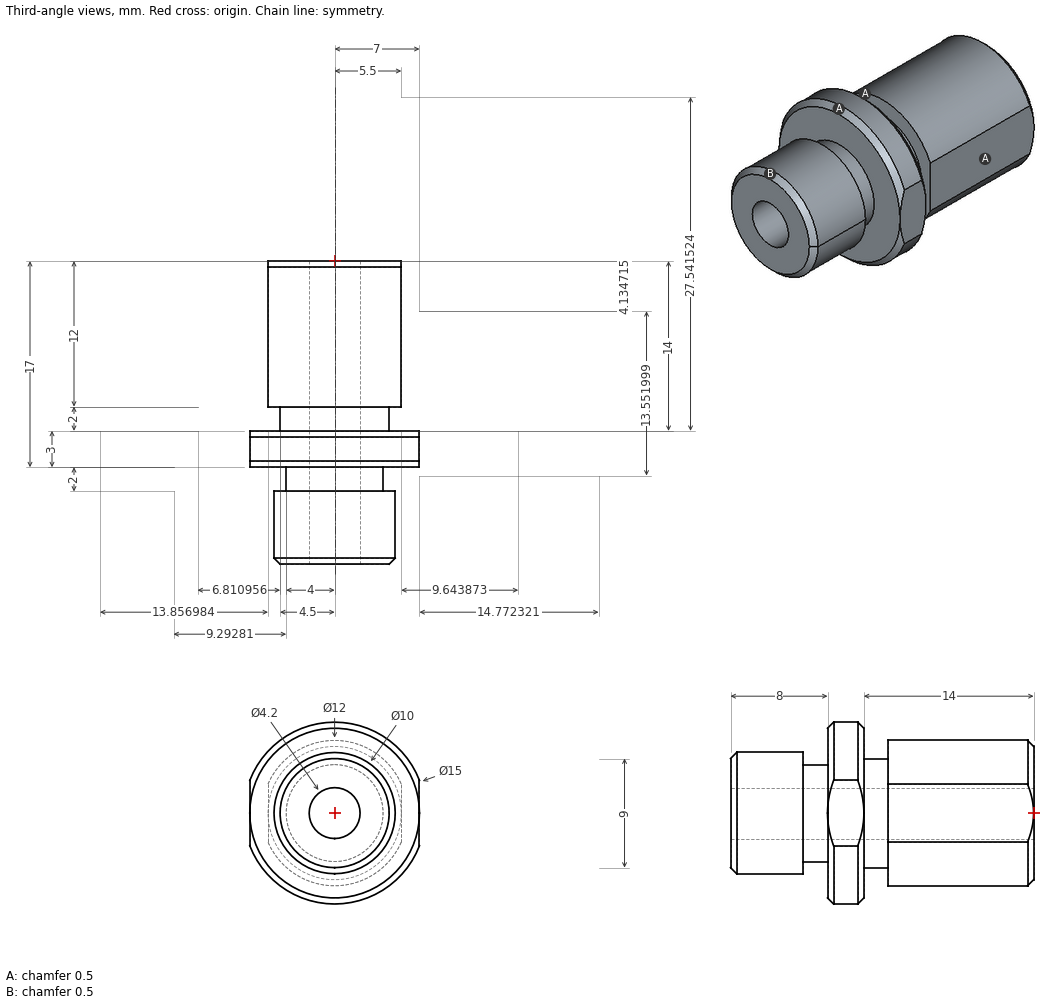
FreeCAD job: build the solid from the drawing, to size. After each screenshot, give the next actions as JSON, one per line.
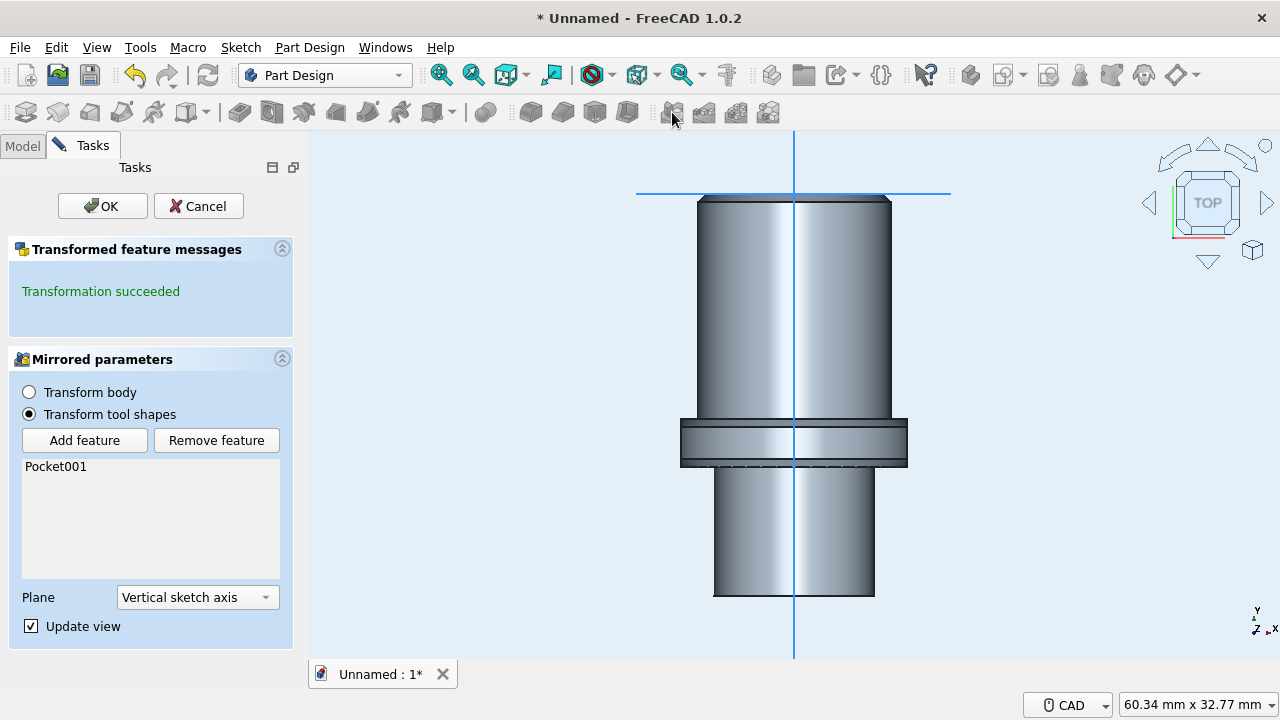
{"action": "left_click", "coordinate": [198, 598]}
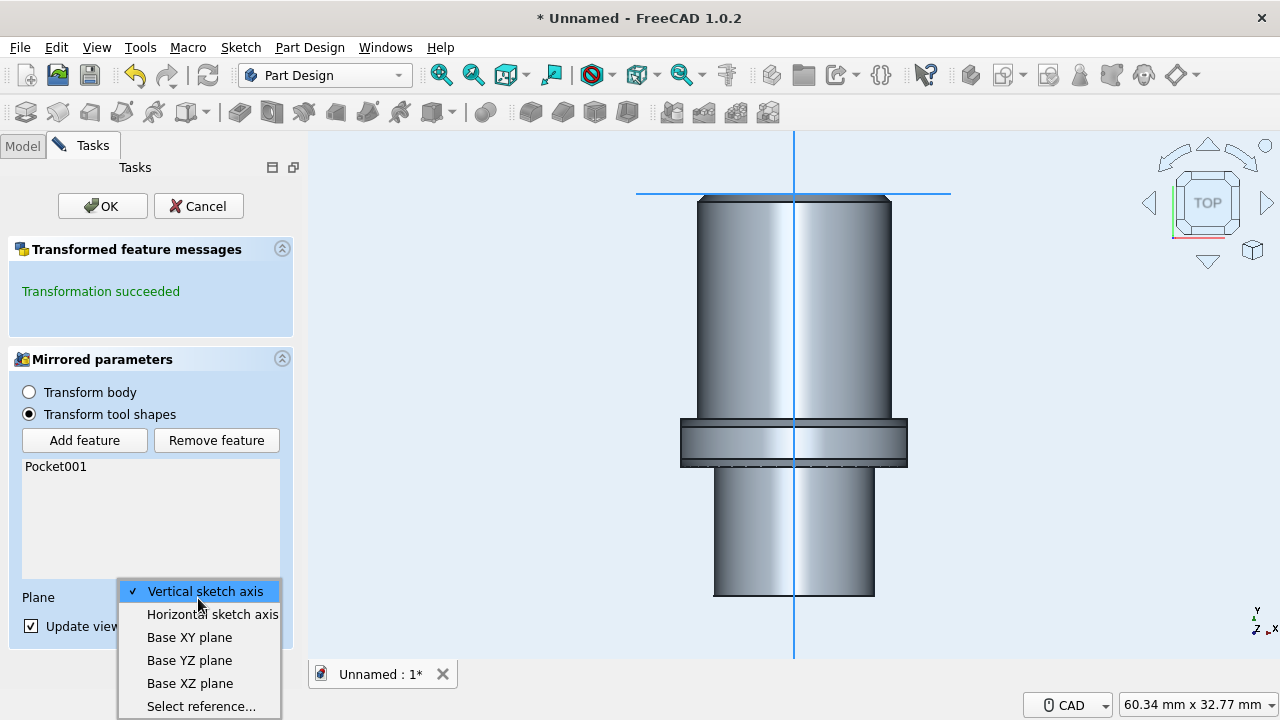
{"action": "left_click", "coordinate": [198, 660]}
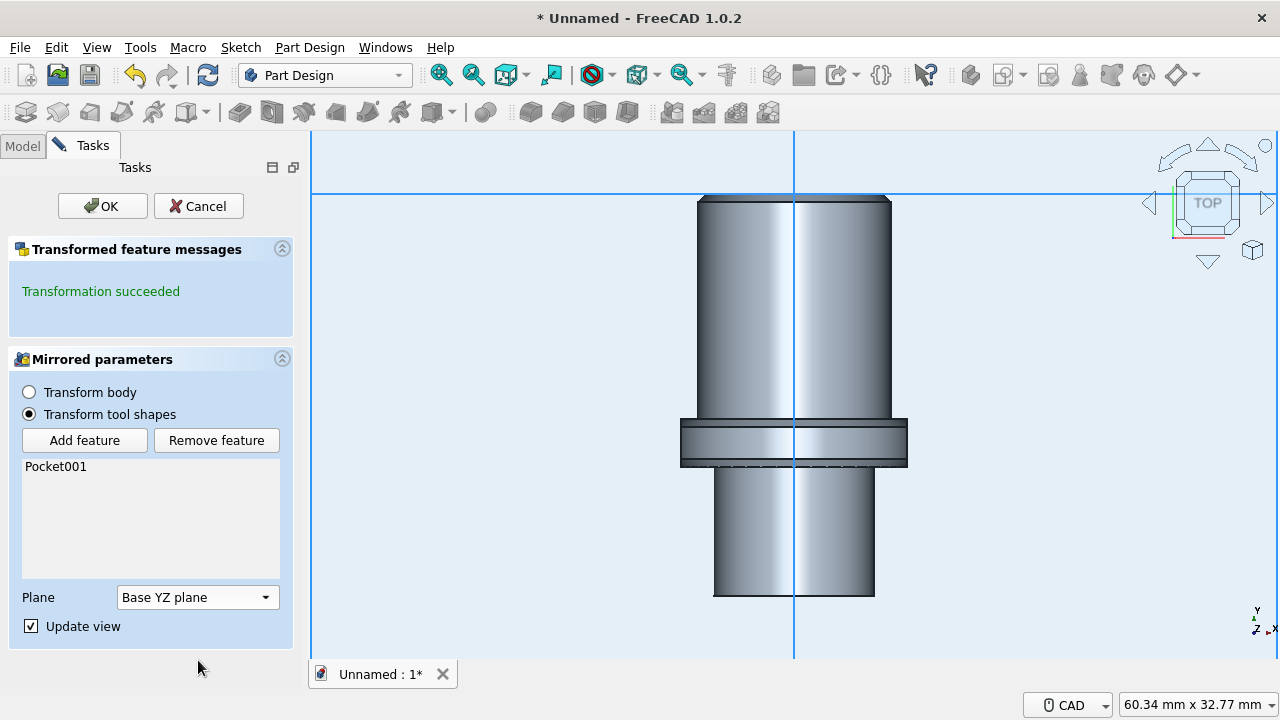
{"action": "left_click", "coordinate": [103, 206]}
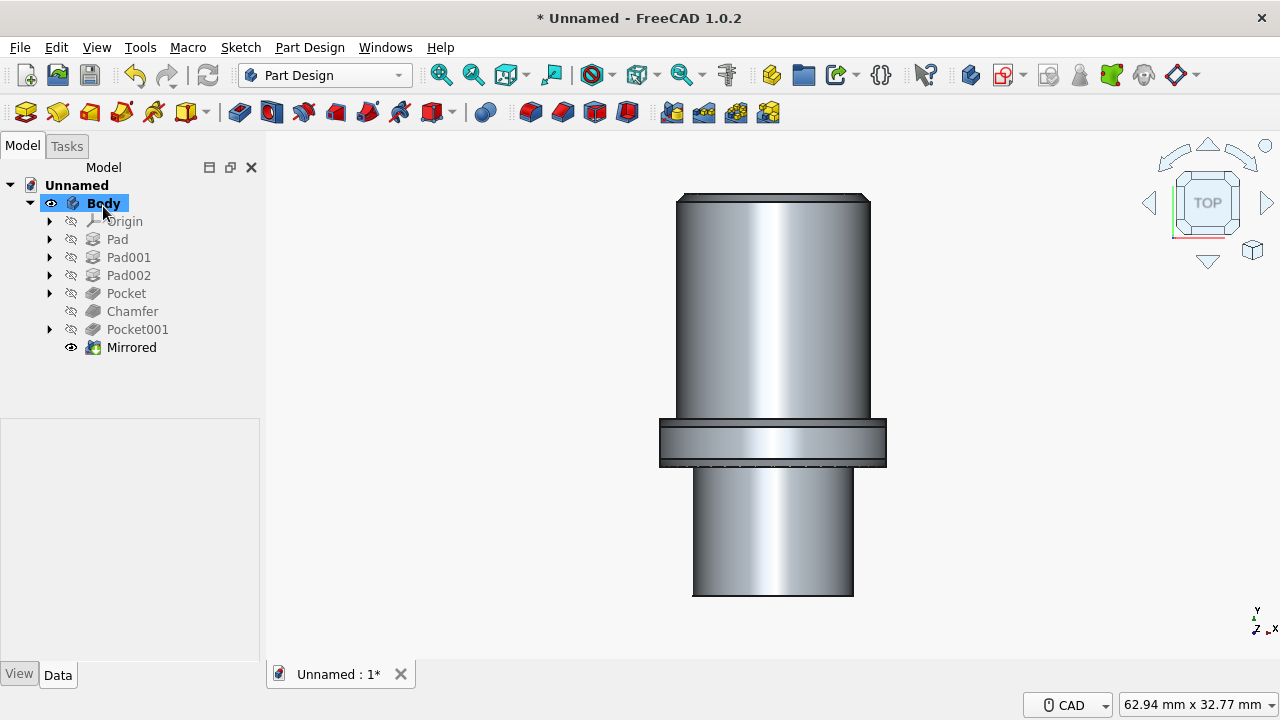
{"action": "left_click", "coordinate": [748, 595]}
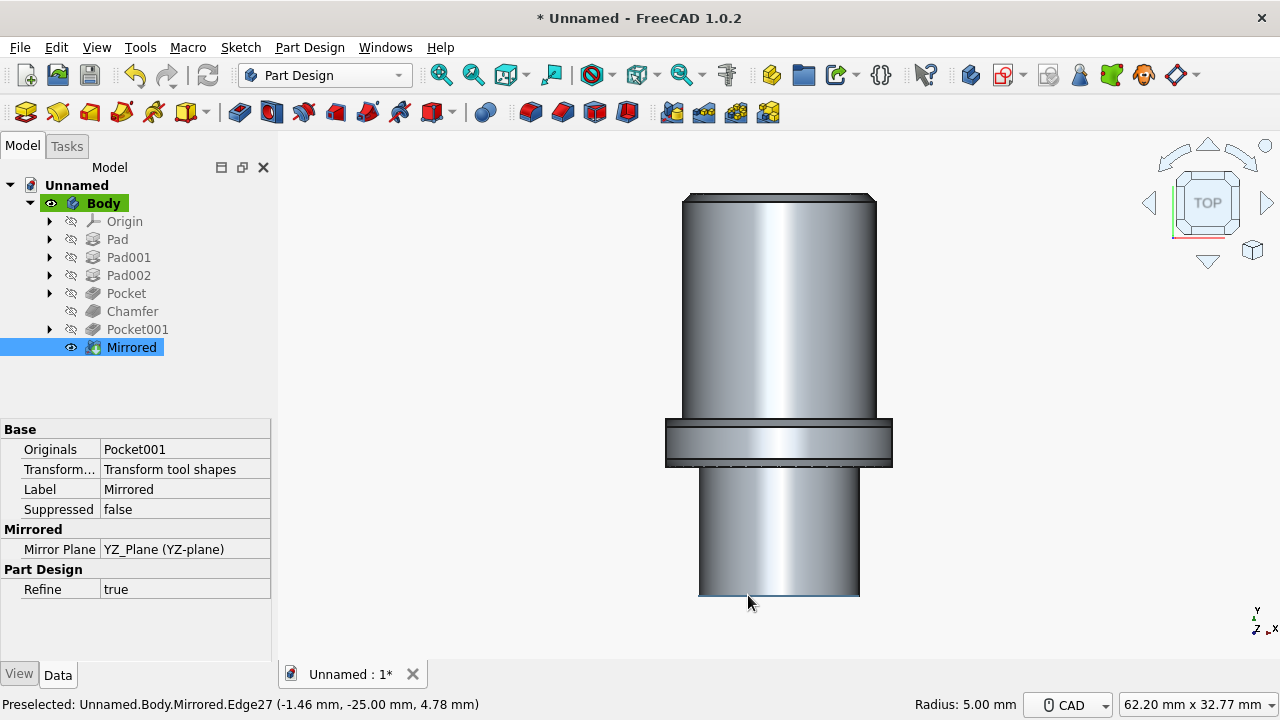
{"action": "left_click", "coordinate": [564, 112]}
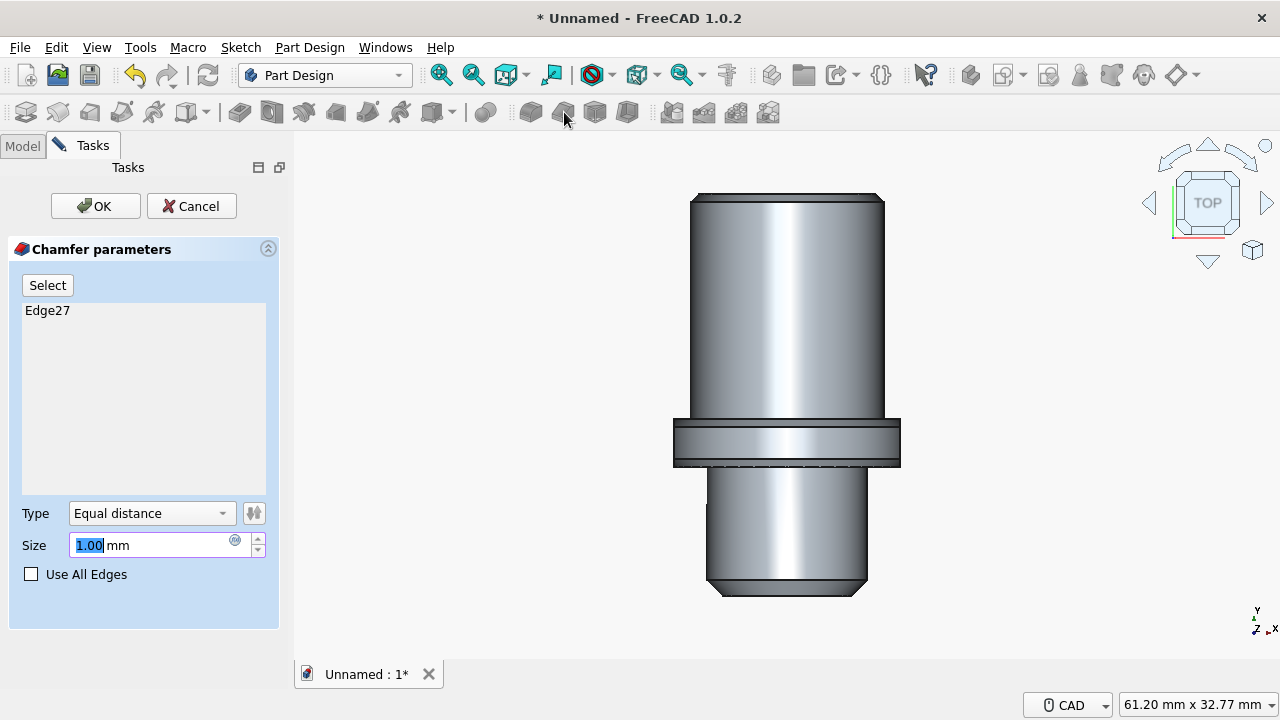
{"action": "type", "text": "0.5"}
{"action": "key", "text": "Tab"}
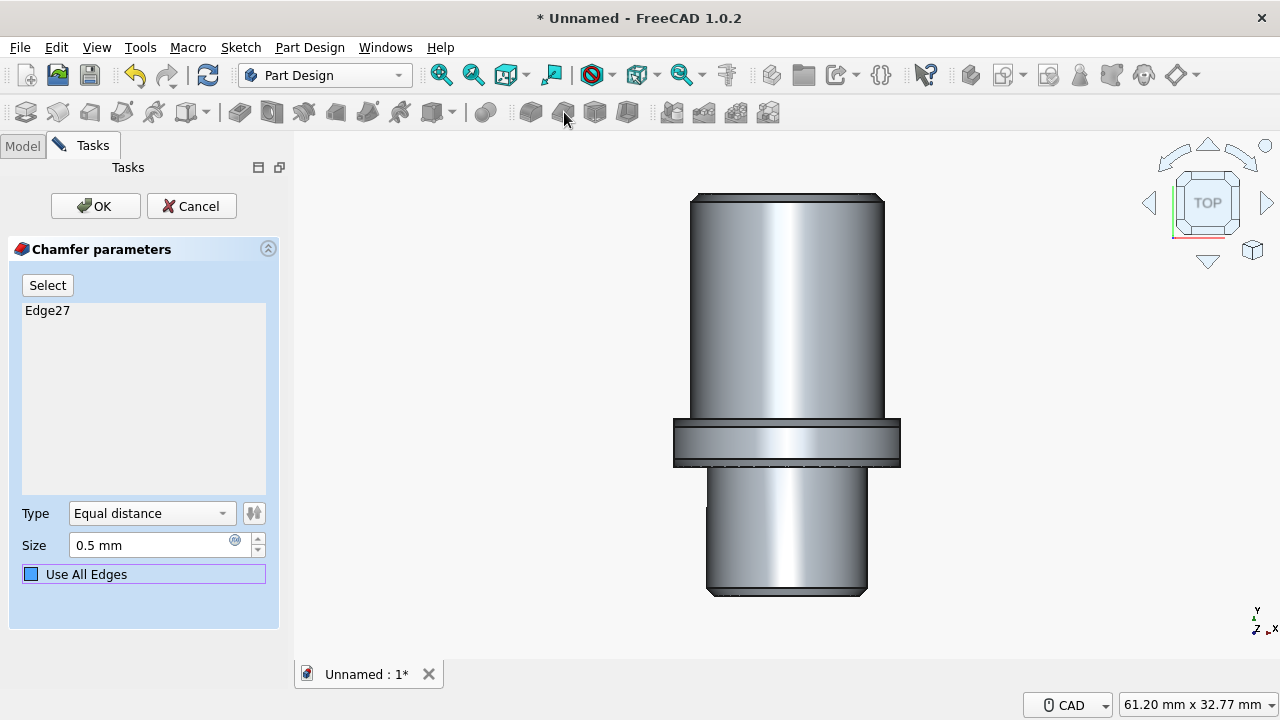
{"action": "left_click", "coordinate": [96, 206]}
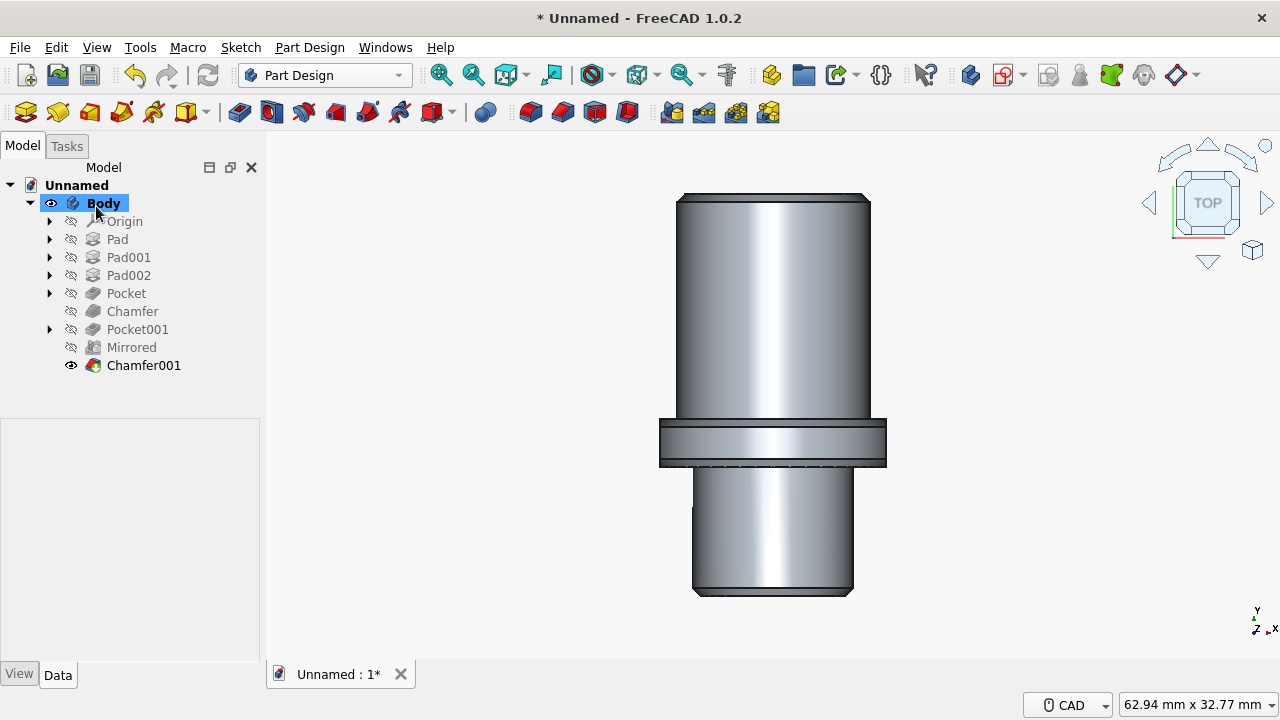
{"action": "left_click", "coordinate": [1004, 76]}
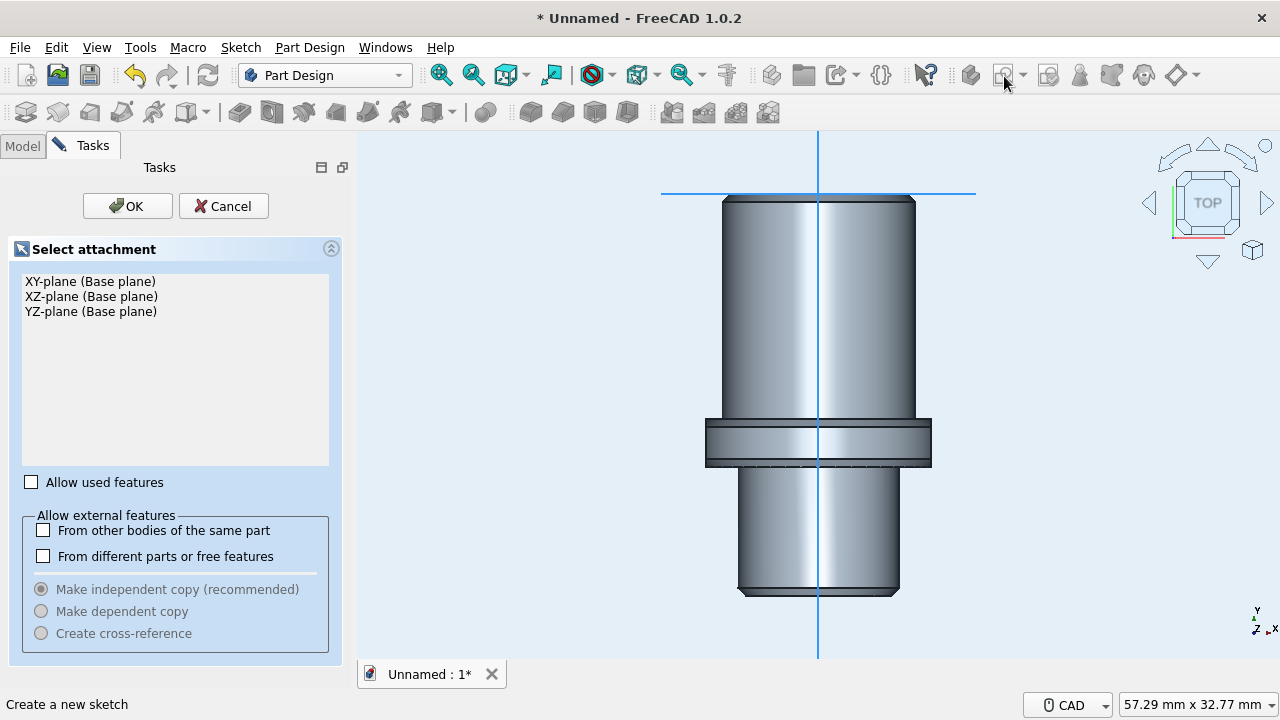
{"action": "left_click", "coordinate": [82, 282]}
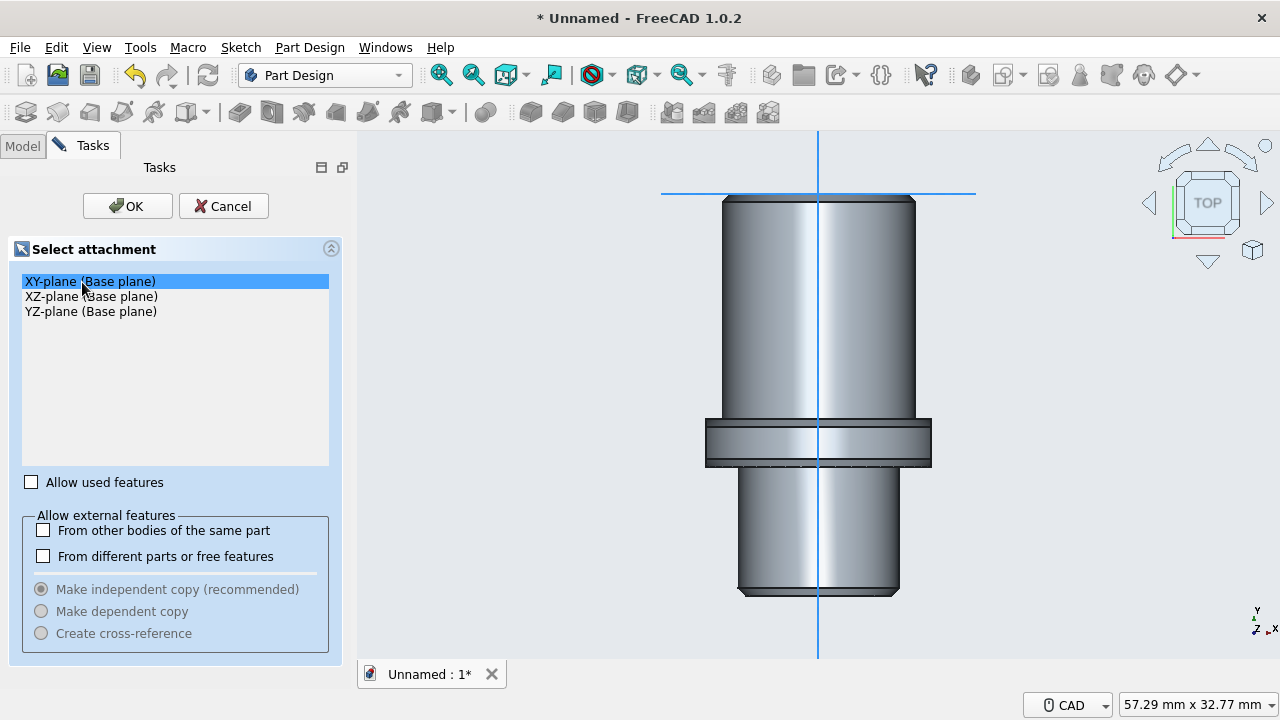
{"action": "left_click", "coordinate": [128, 206]}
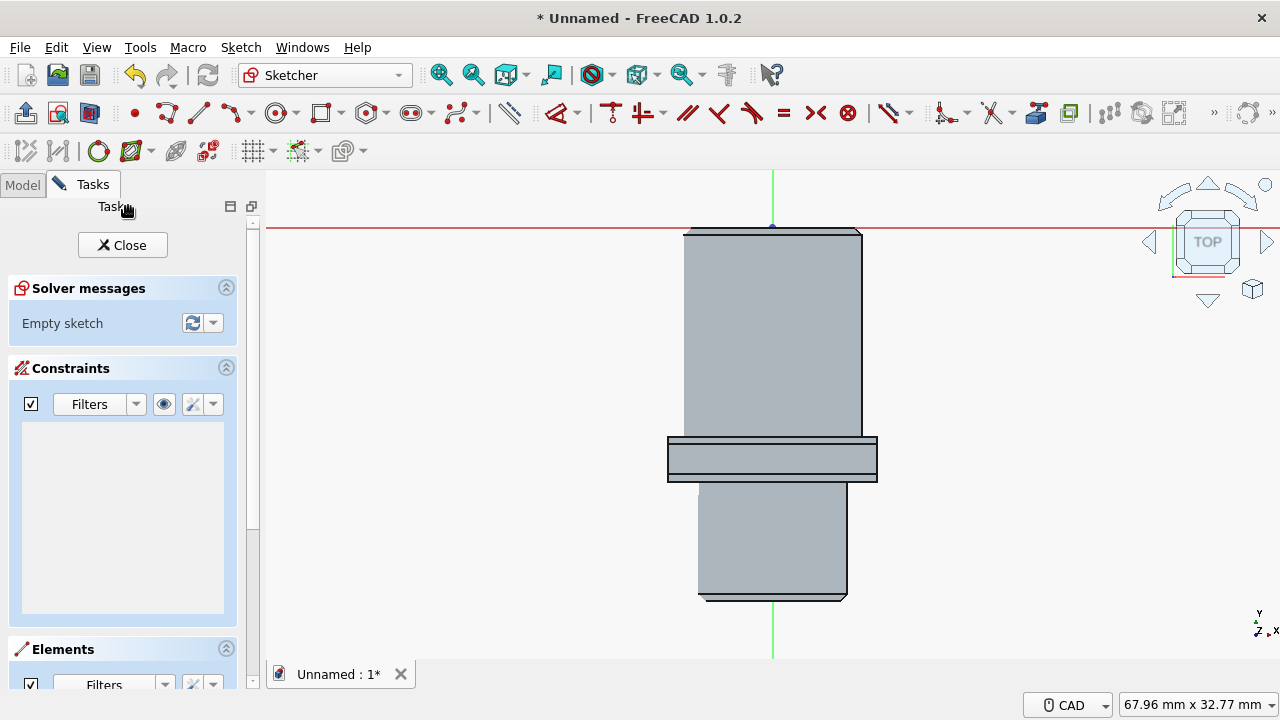
{"action": "key", "text": "q s"}